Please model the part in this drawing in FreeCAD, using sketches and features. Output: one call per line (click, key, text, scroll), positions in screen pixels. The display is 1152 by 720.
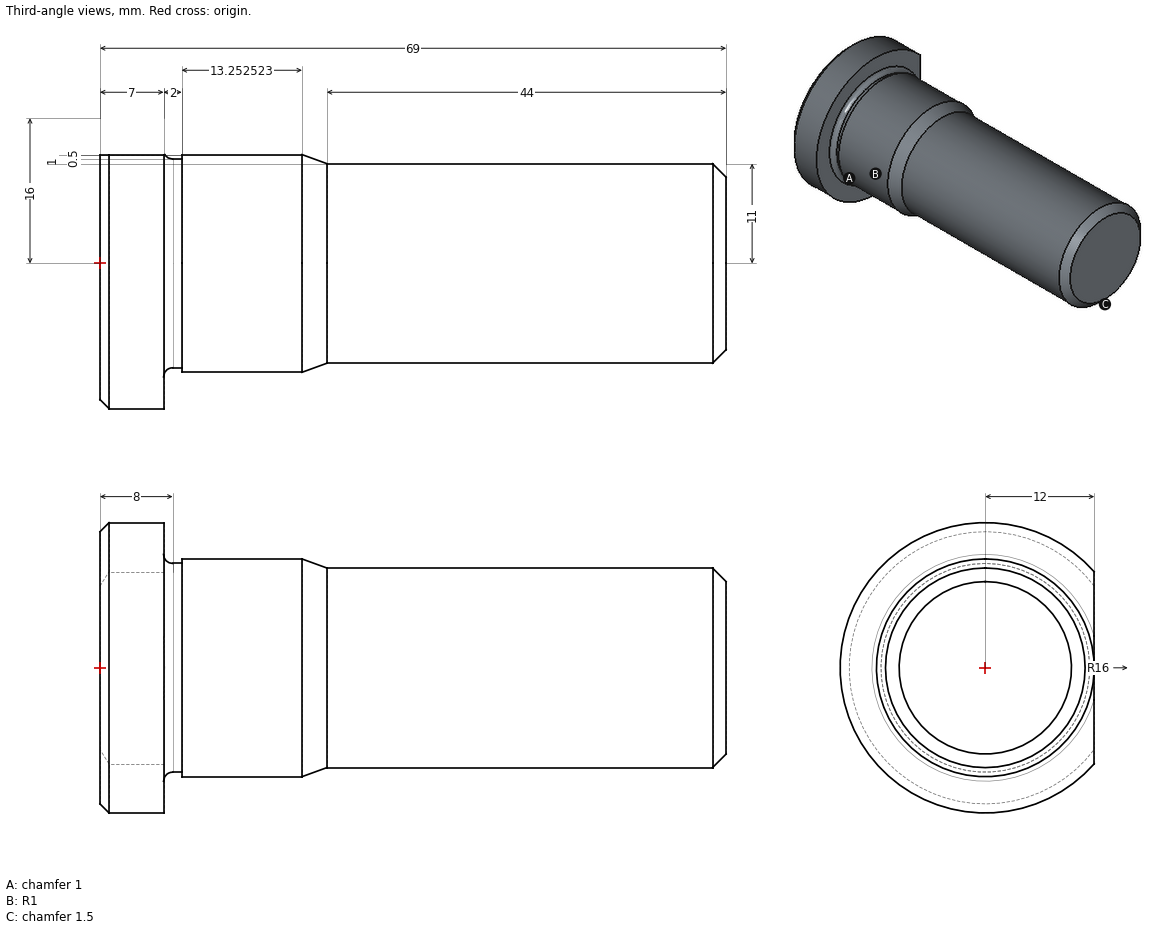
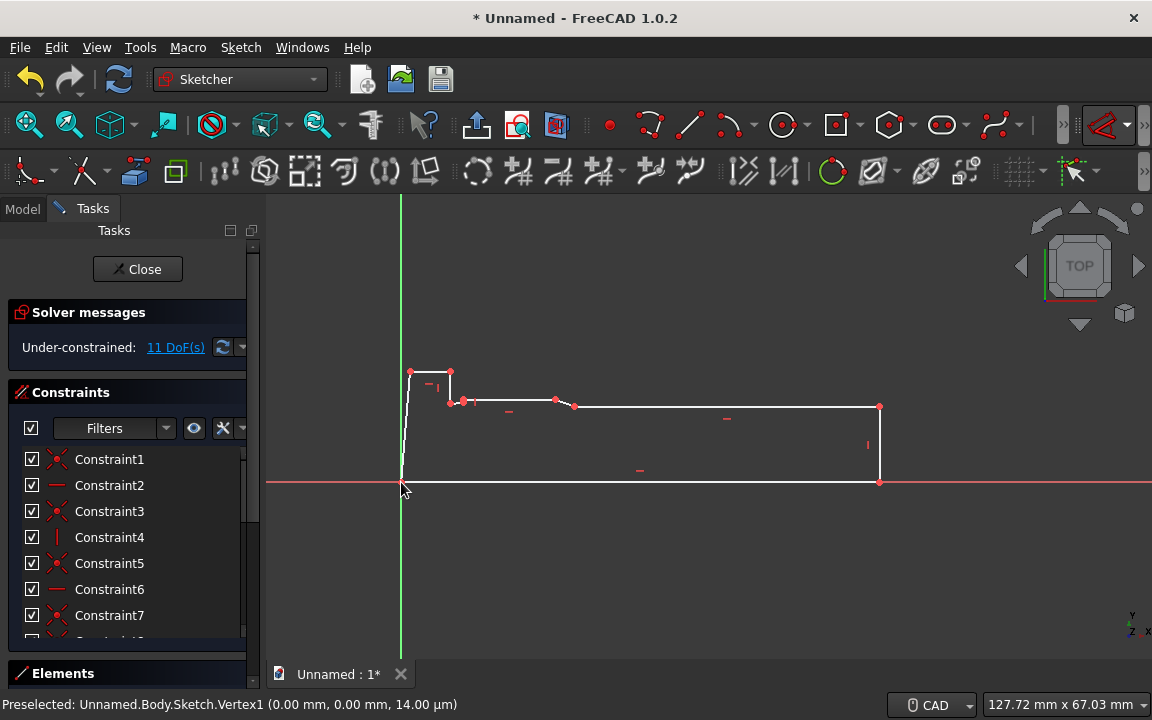
scroll(457, 403, up, 4)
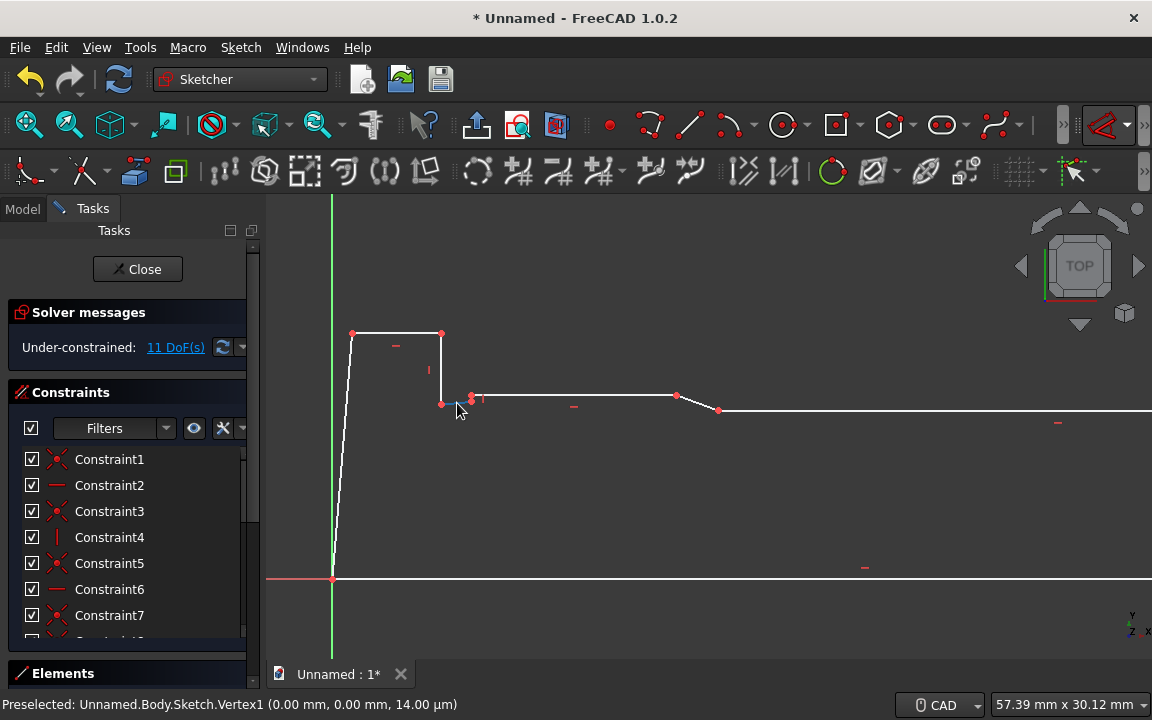
click(457, 403)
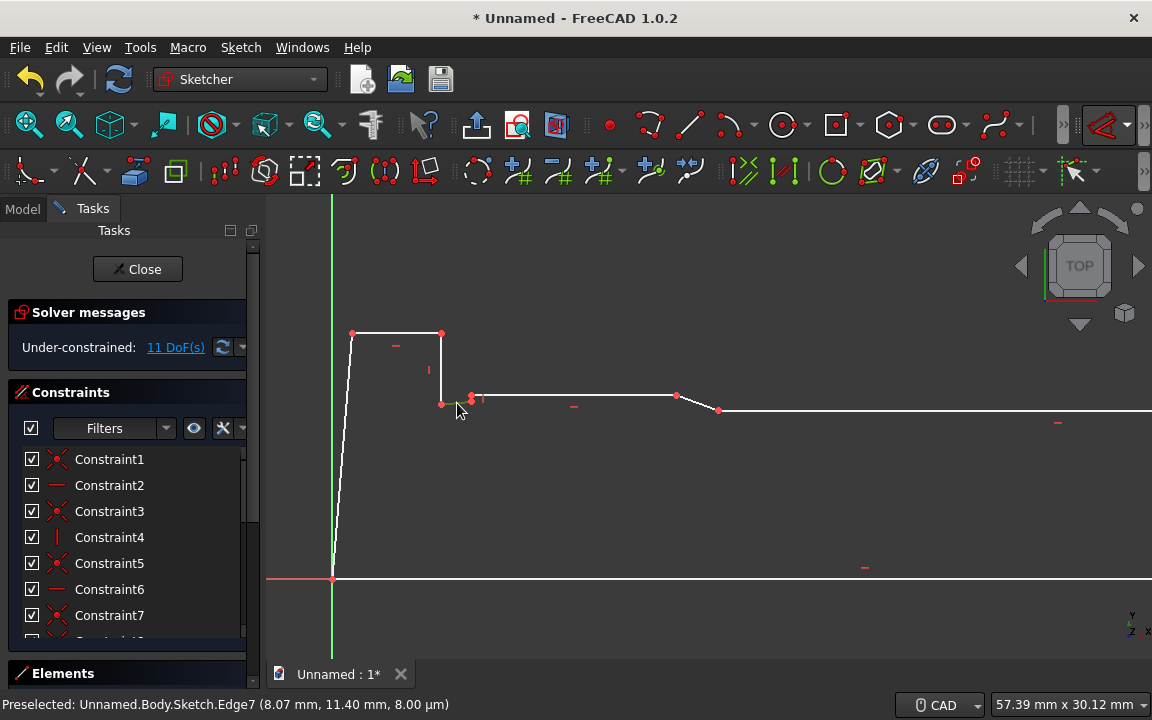
key(h)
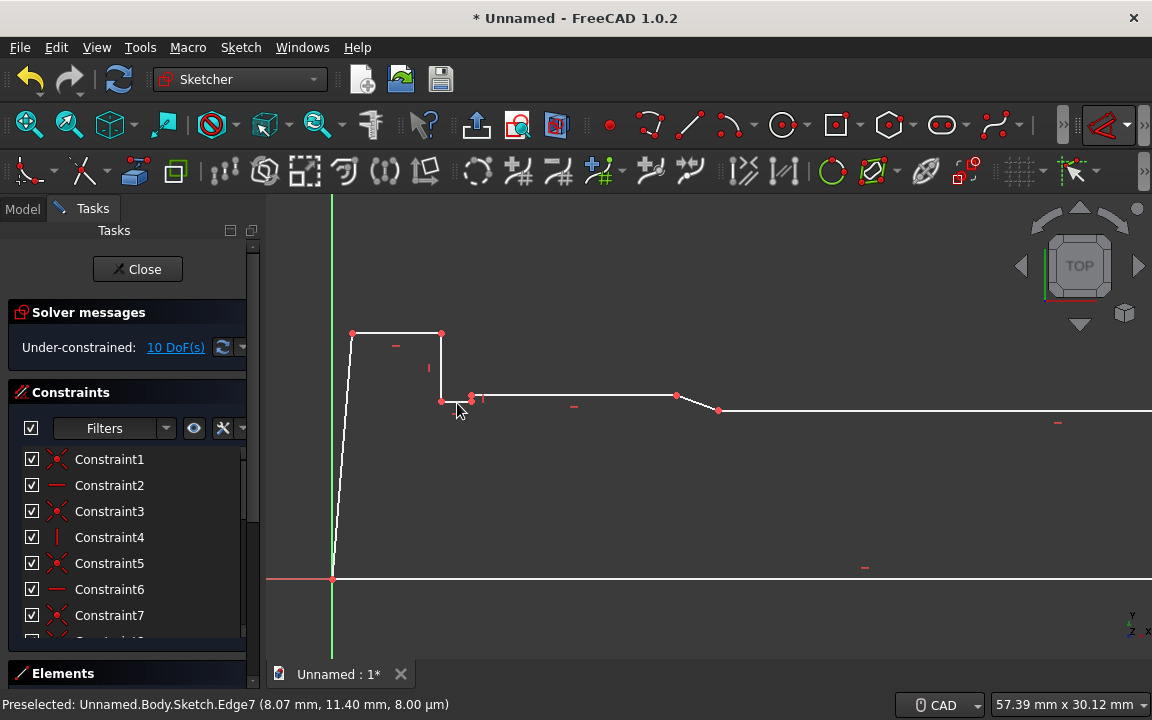
click(346, 407)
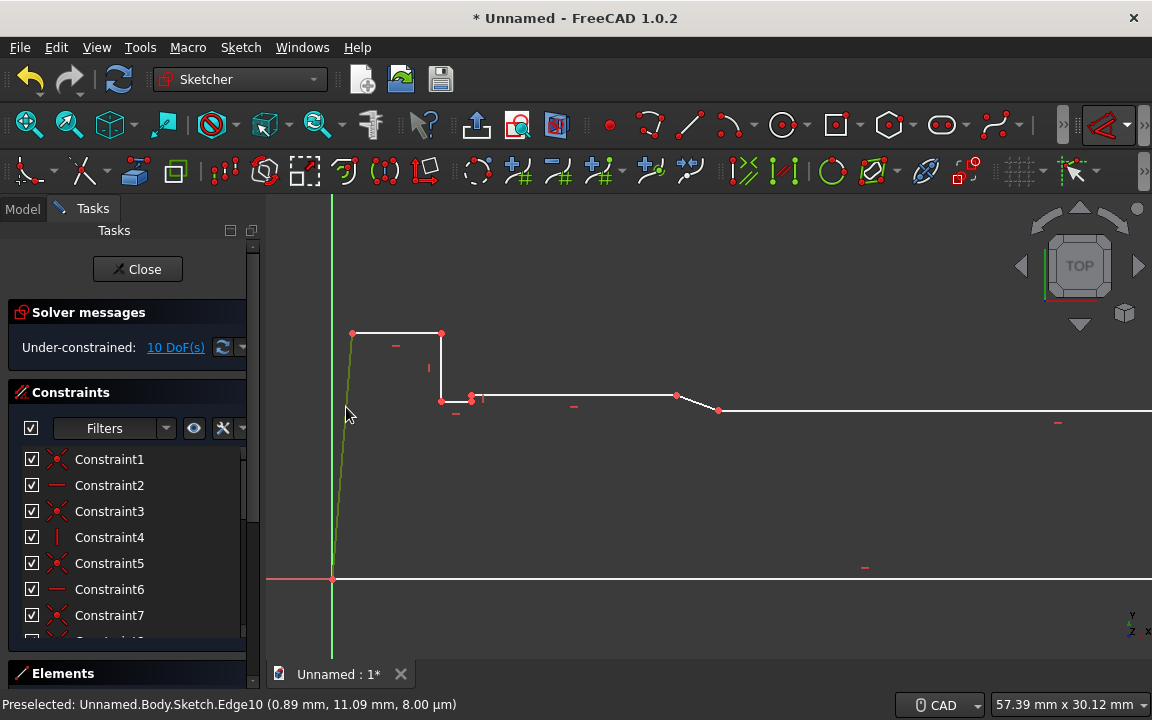
key(v)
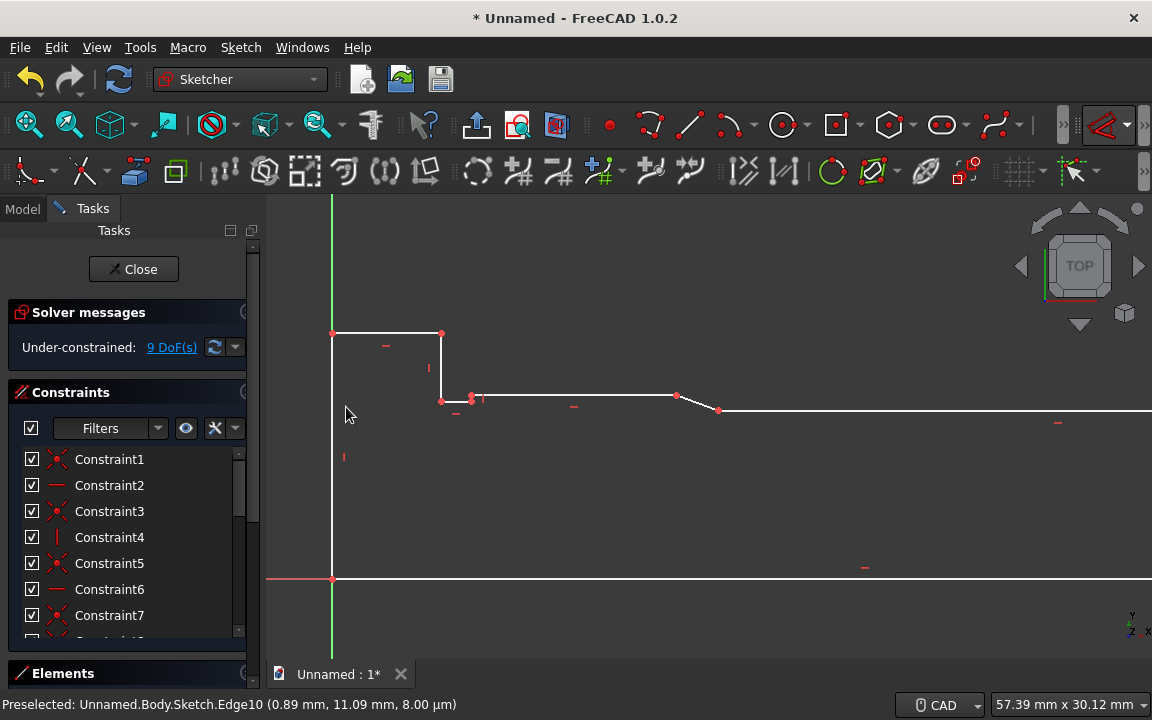
key(d)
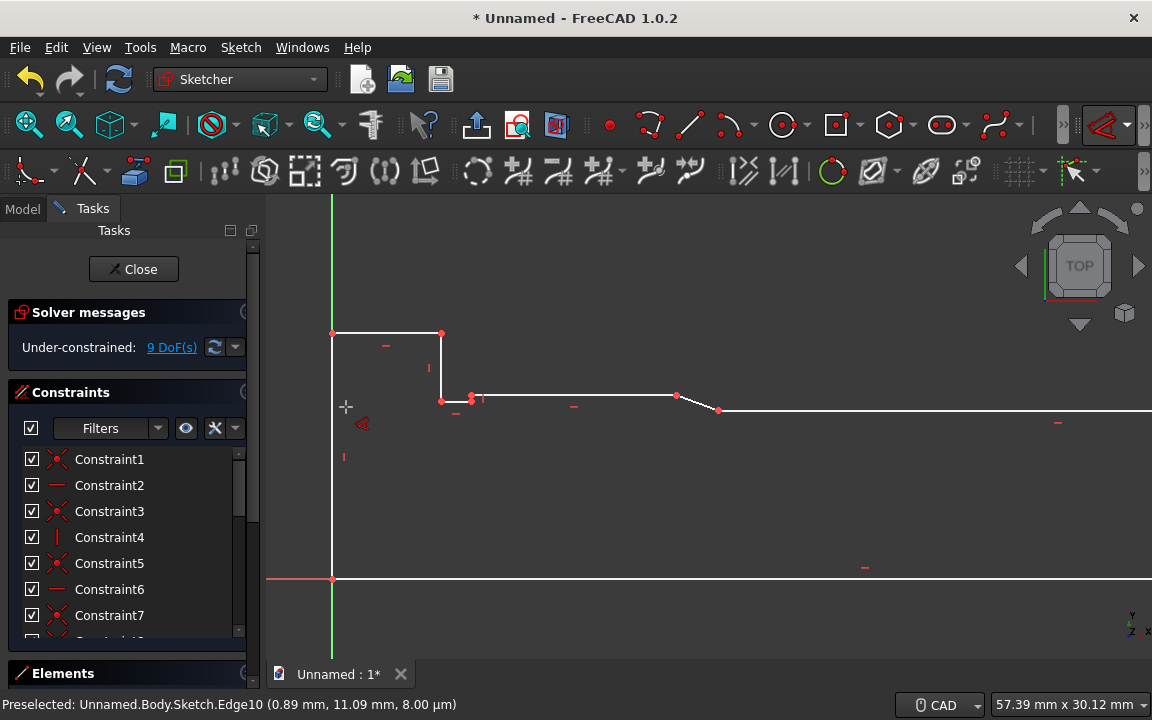
scroll(463, 402, up, 3)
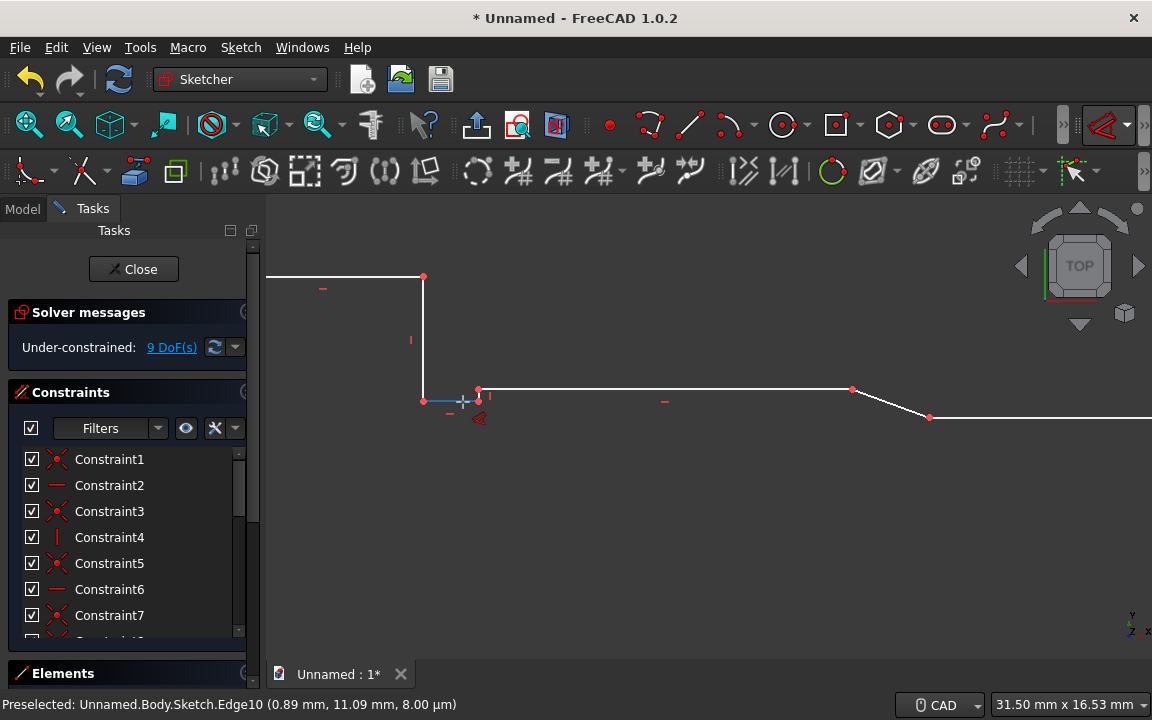
click(462, 401)
click(451, 367)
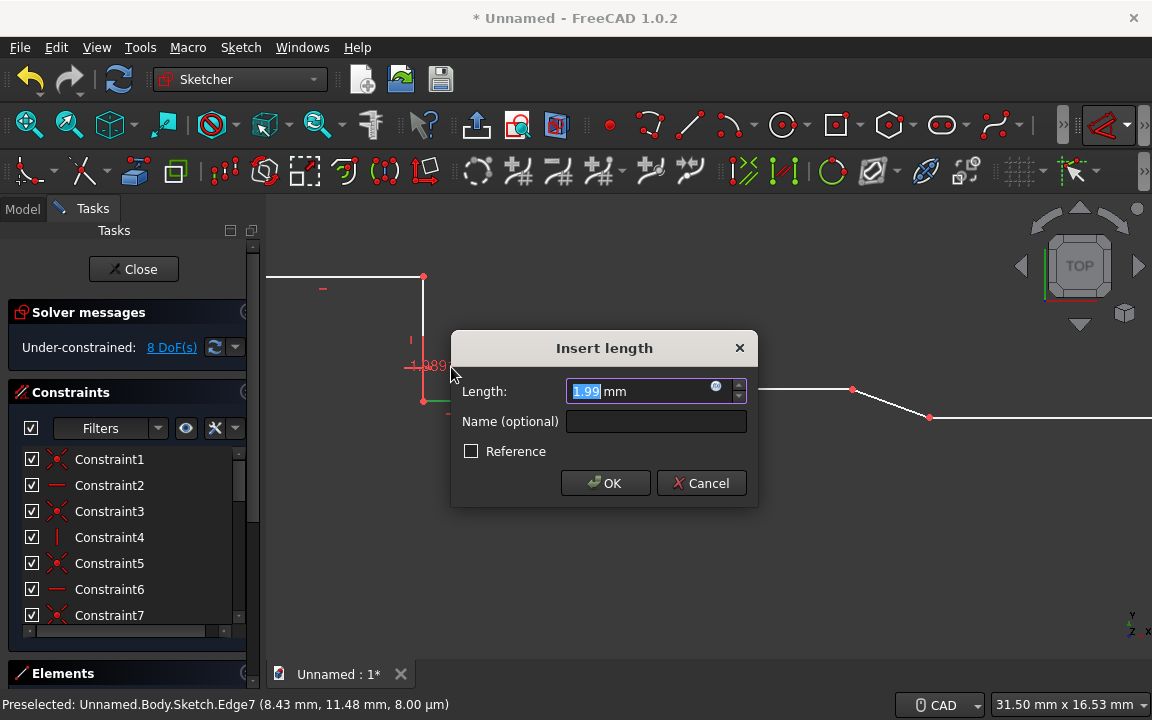
text(2)
key(Return)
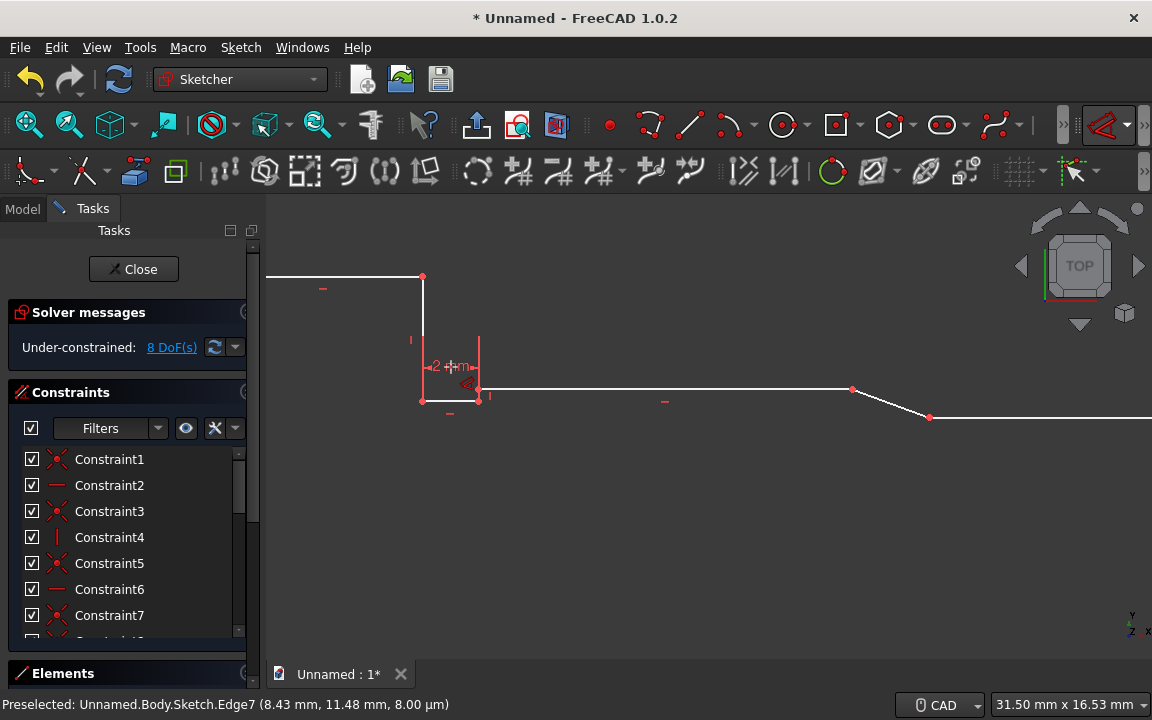
scroll(459, 403, down, 7)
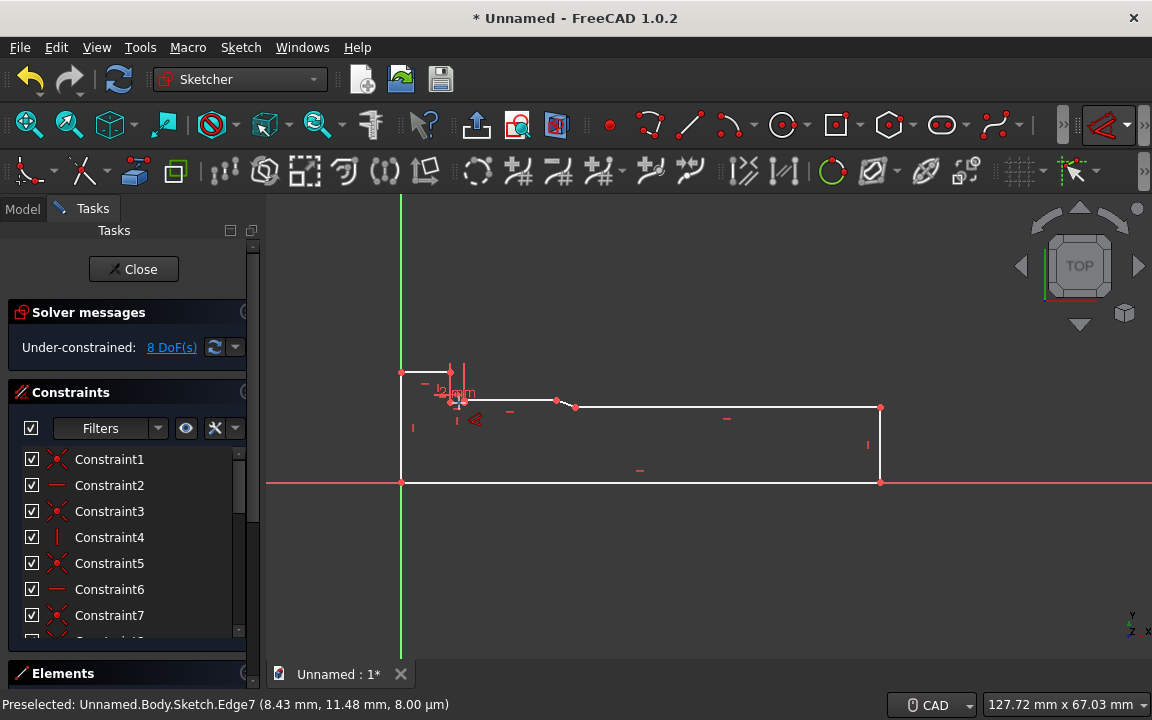
click(436, 372)
click(426, 338)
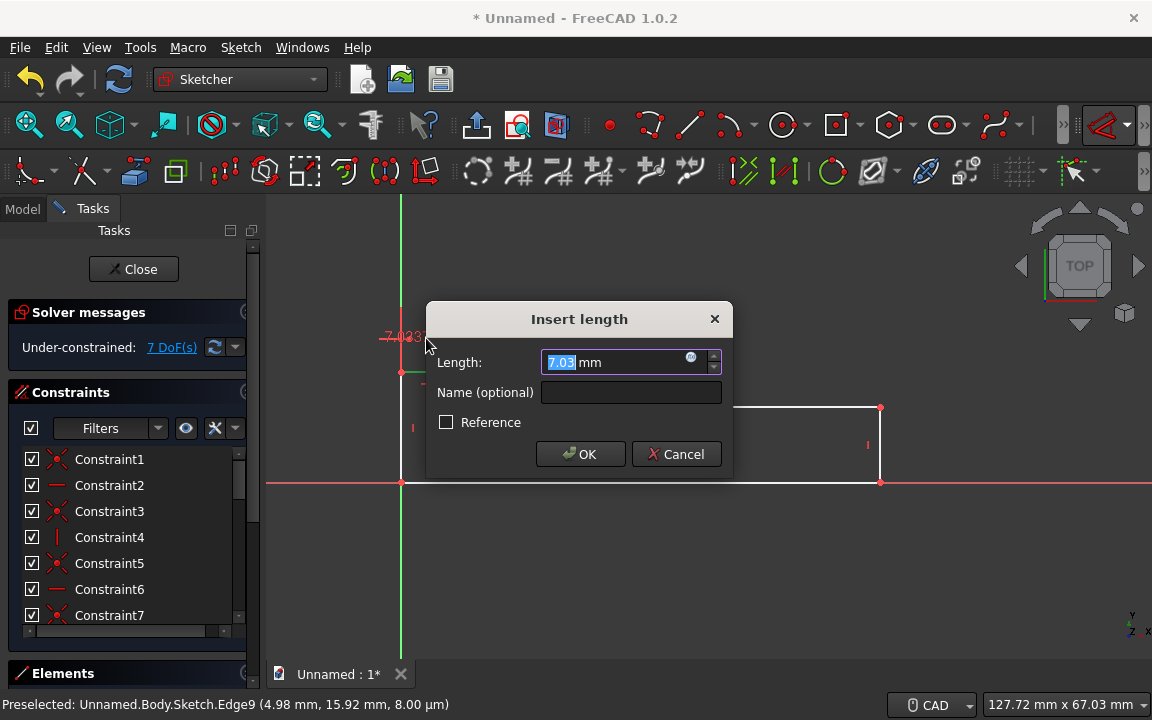
text(7)
key(Return)